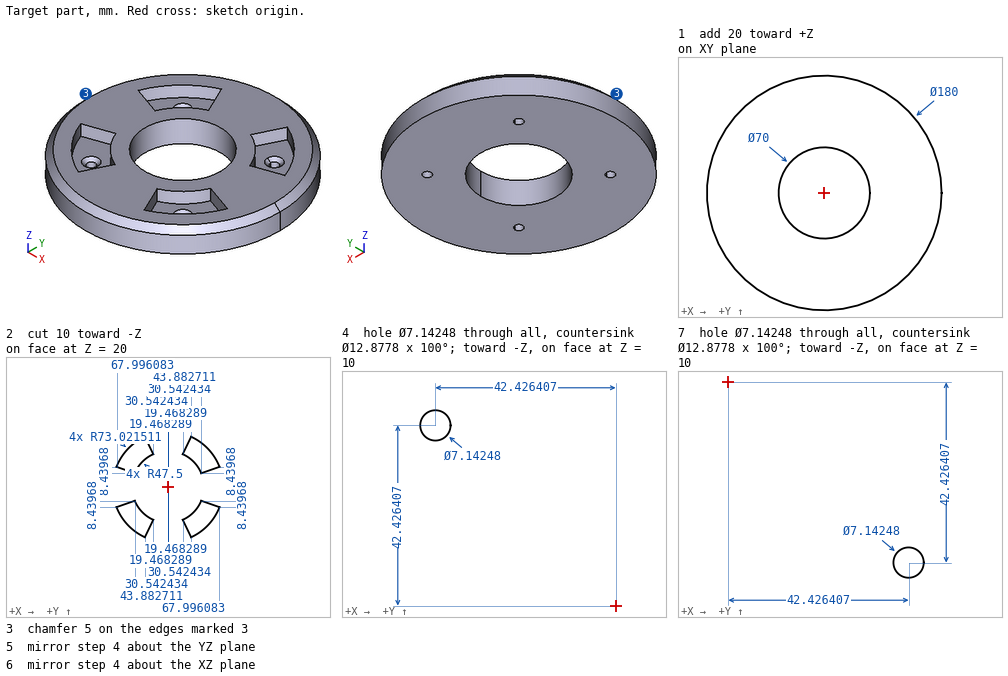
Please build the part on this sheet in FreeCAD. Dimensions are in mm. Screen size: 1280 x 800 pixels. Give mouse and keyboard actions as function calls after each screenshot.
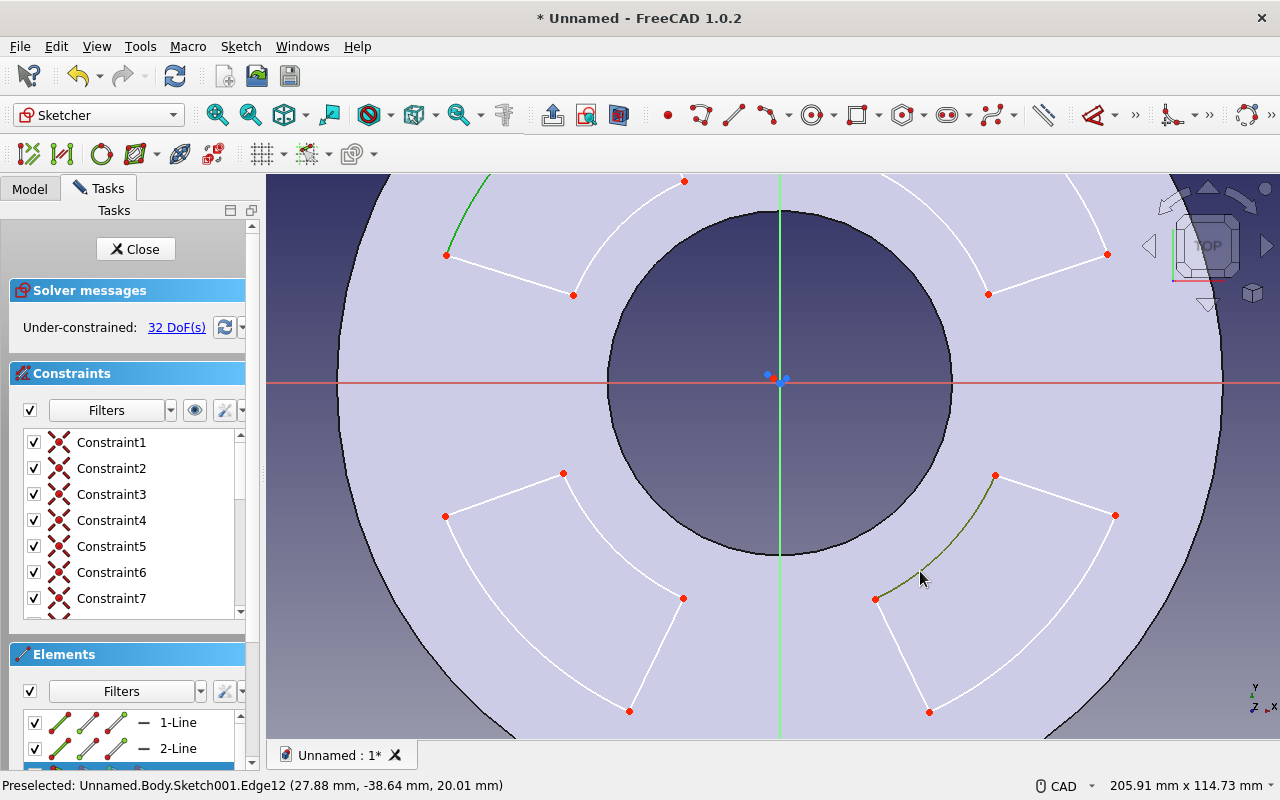
key(c)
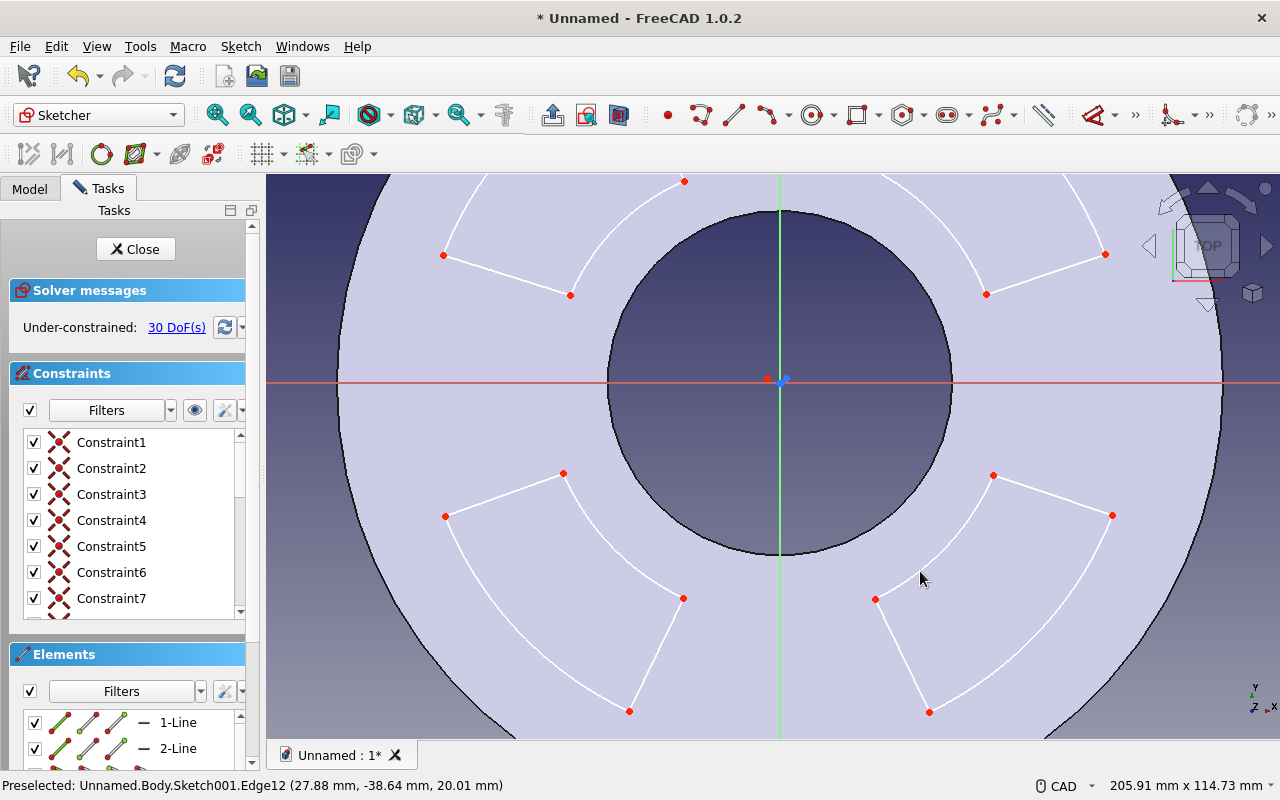
click(467, 205)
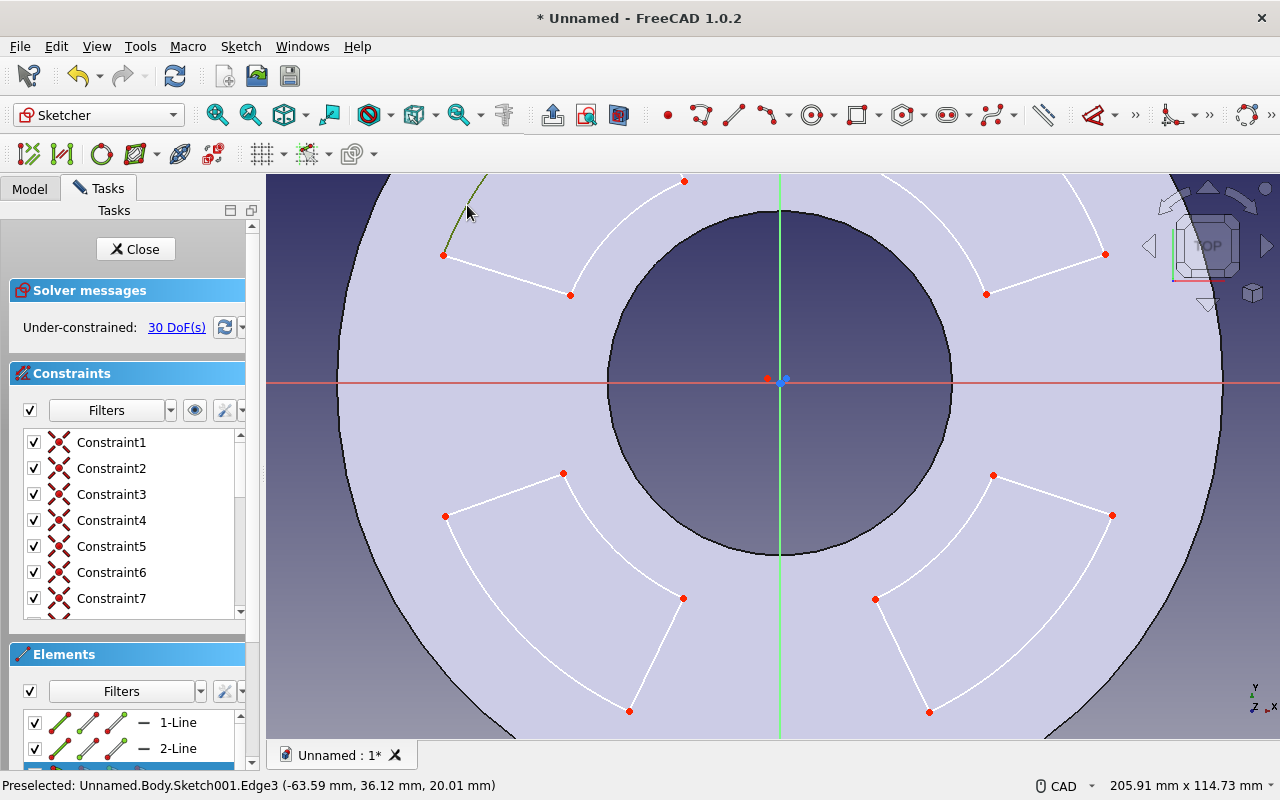
click(484, 589)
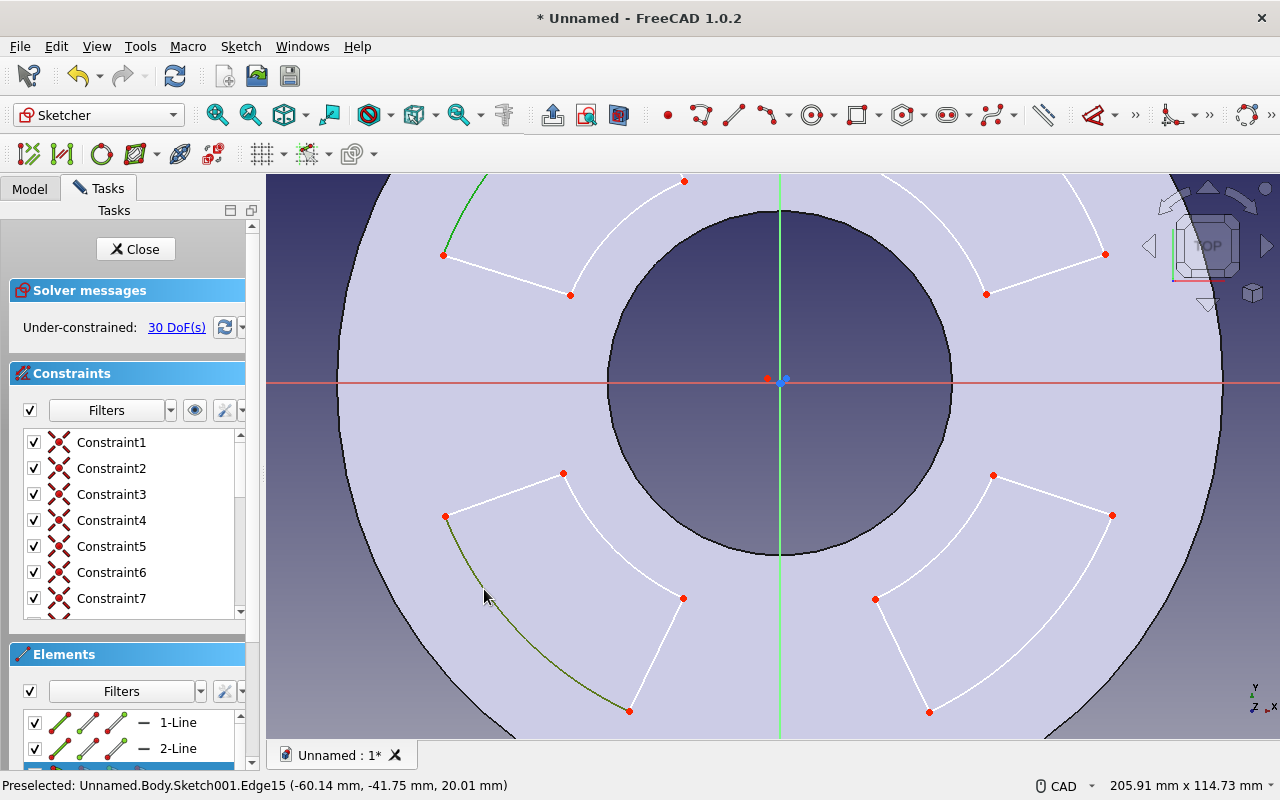
key(c)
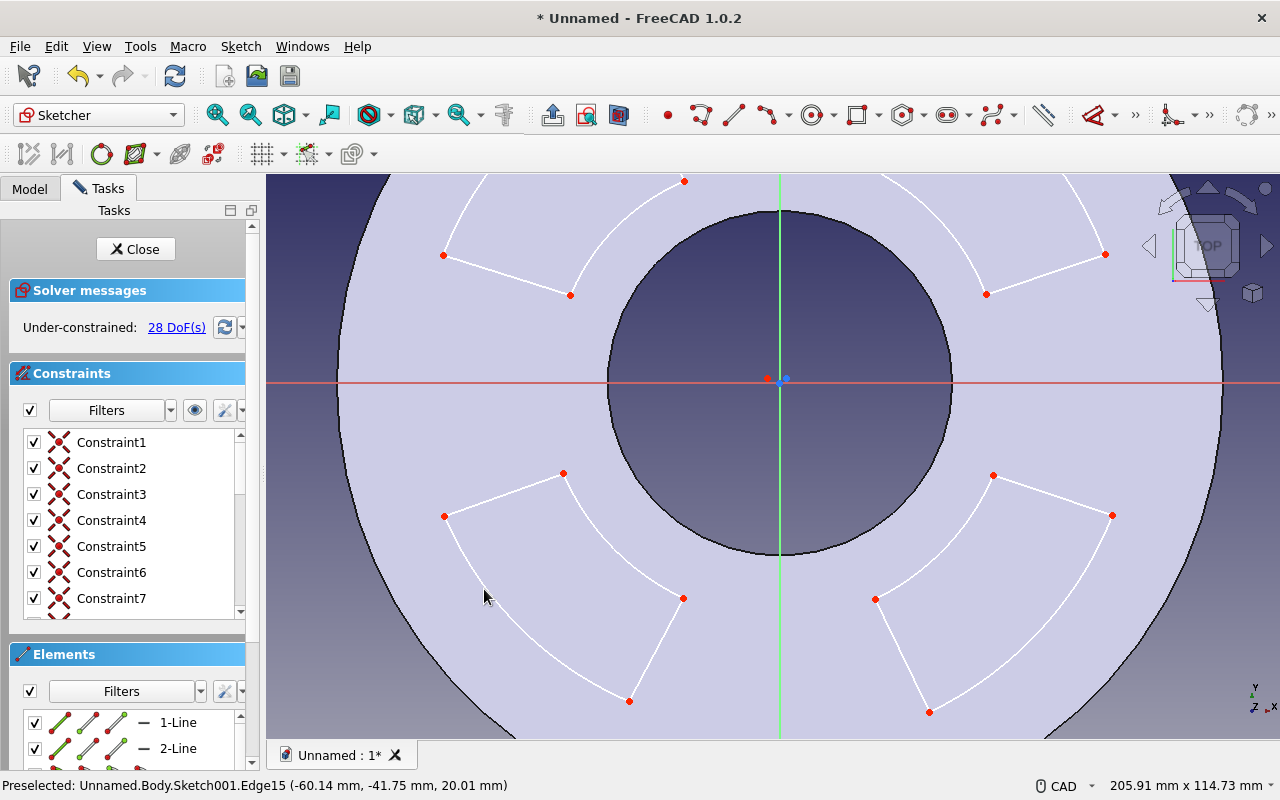
click(467, 205)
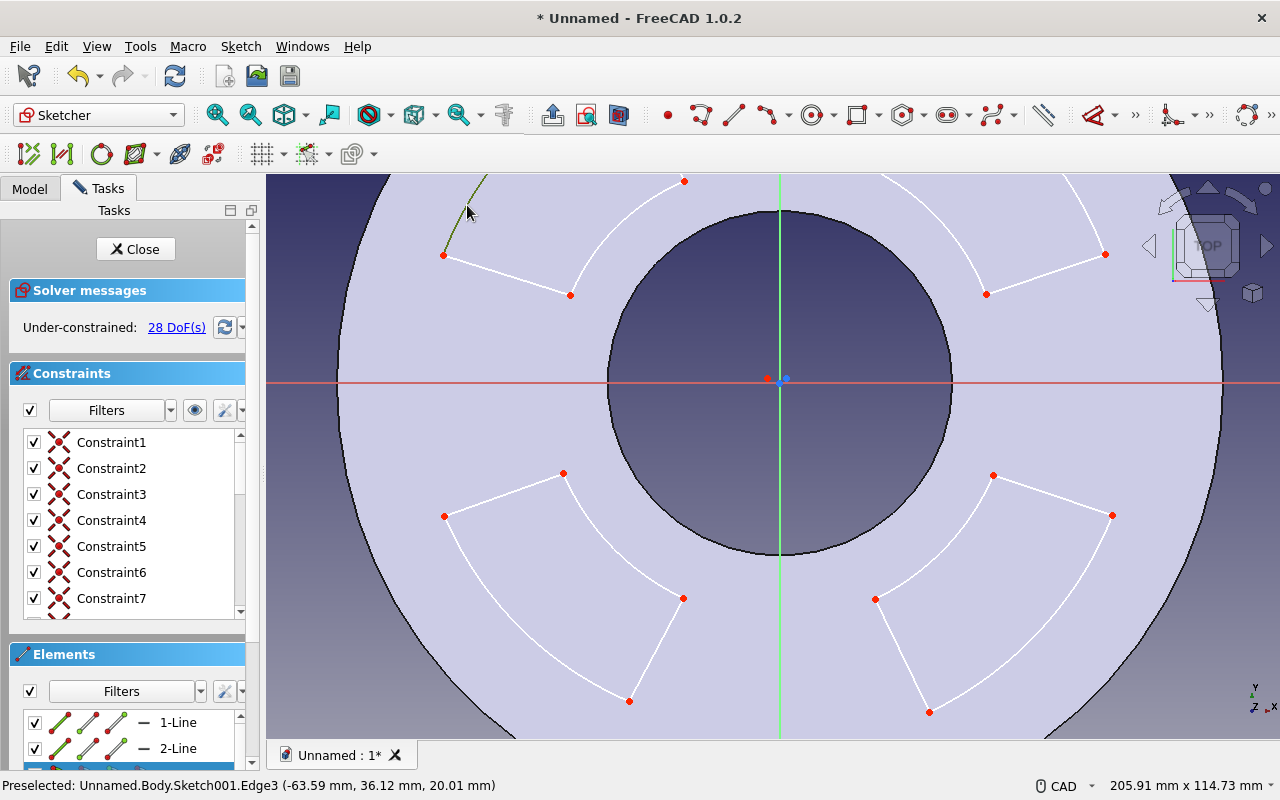
click(589, 520)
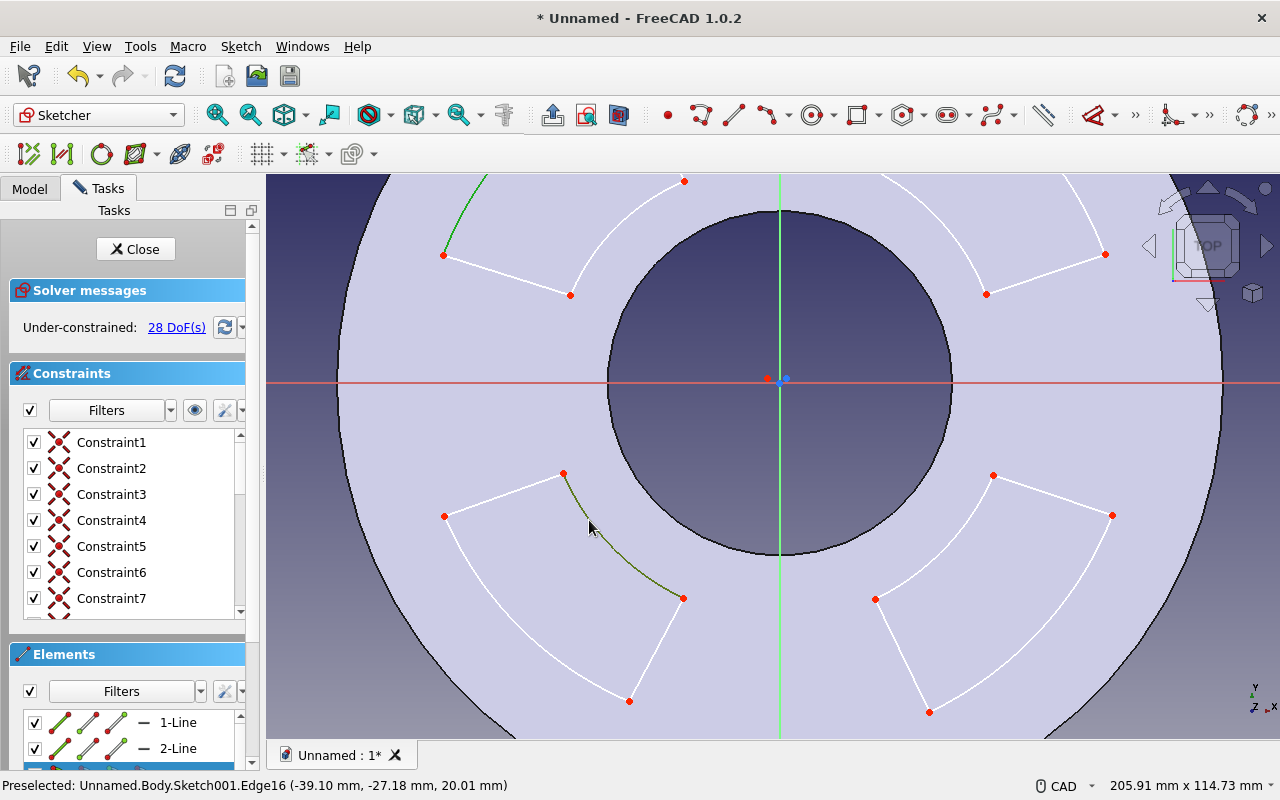
key(c)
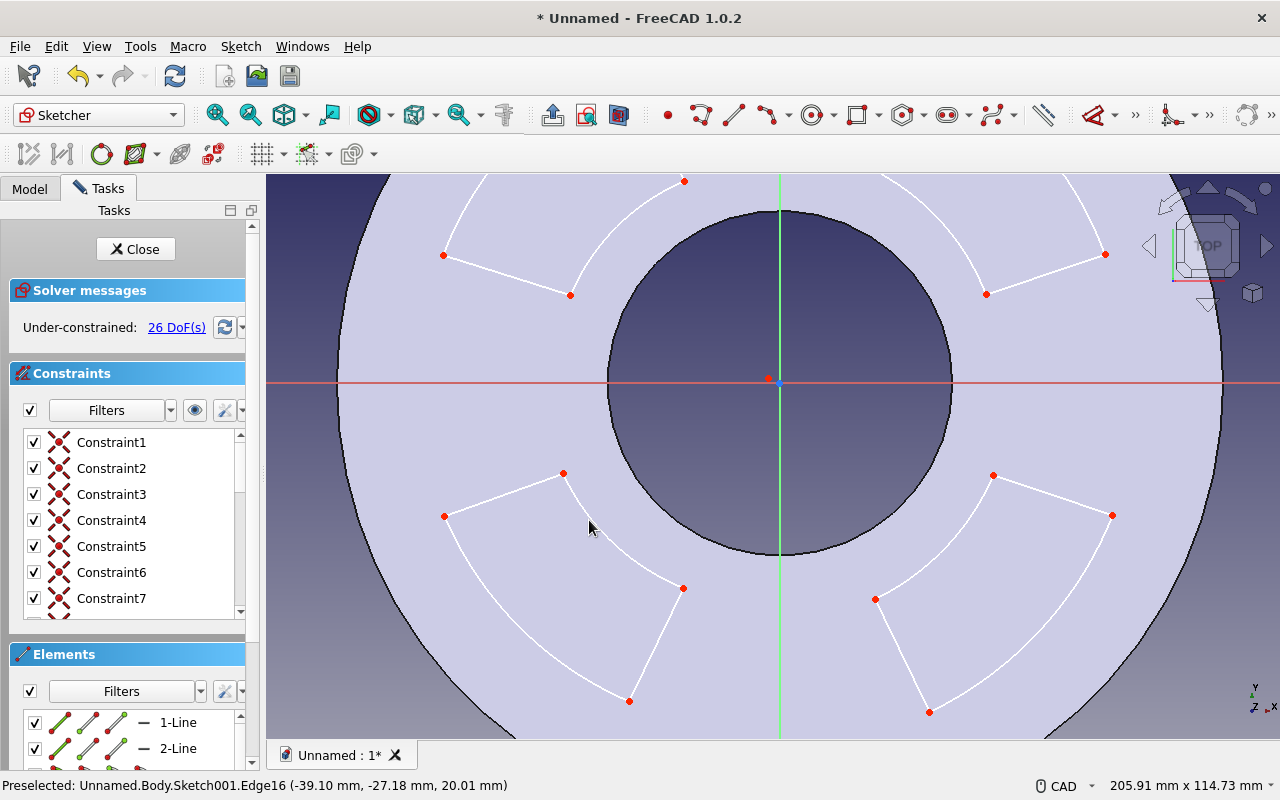
drag(758, 368, 790, 393)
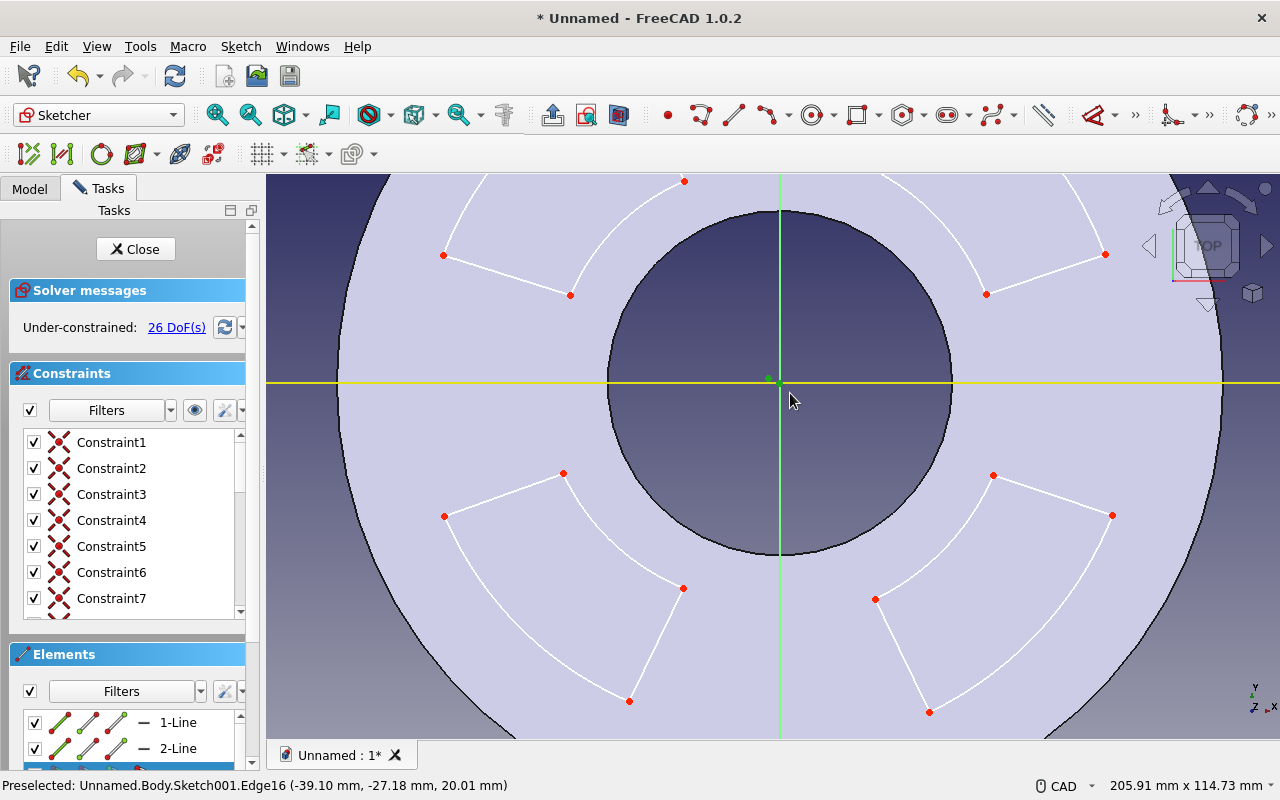
key(c)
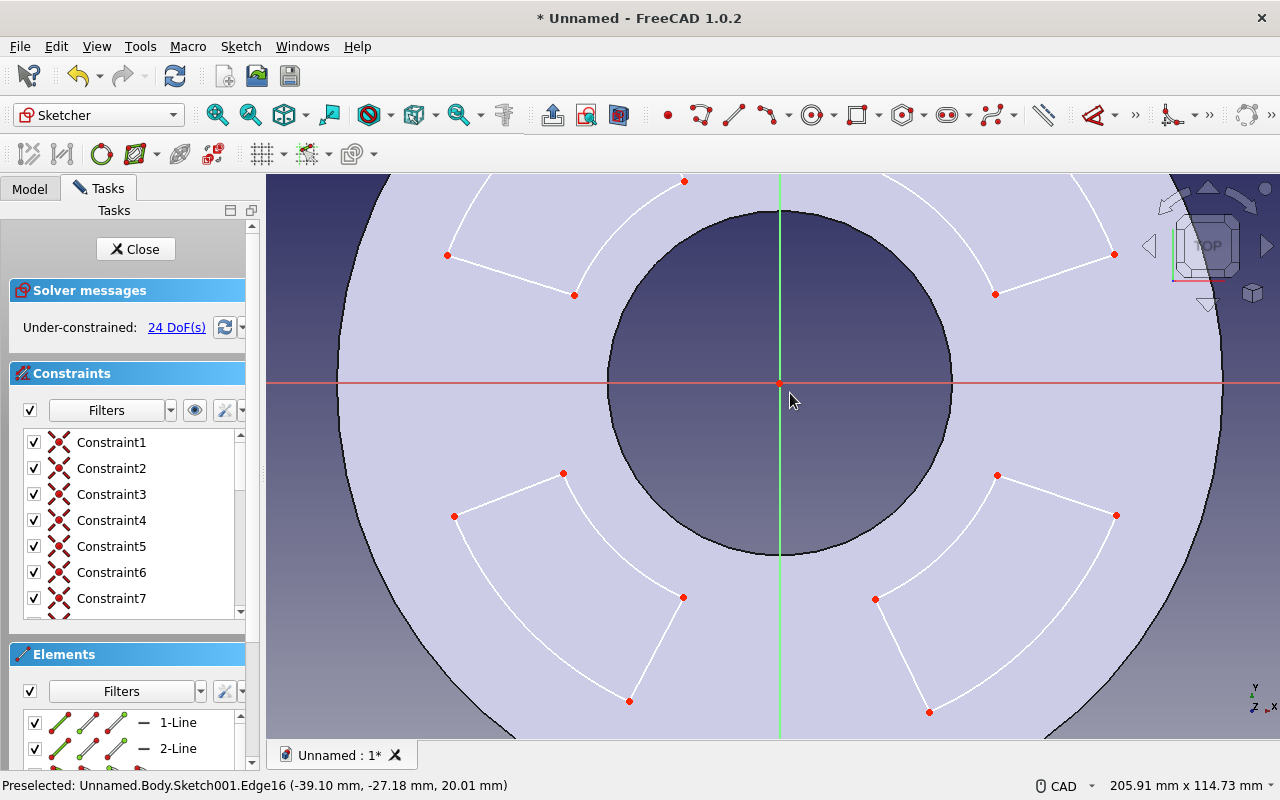
click(470, 206)